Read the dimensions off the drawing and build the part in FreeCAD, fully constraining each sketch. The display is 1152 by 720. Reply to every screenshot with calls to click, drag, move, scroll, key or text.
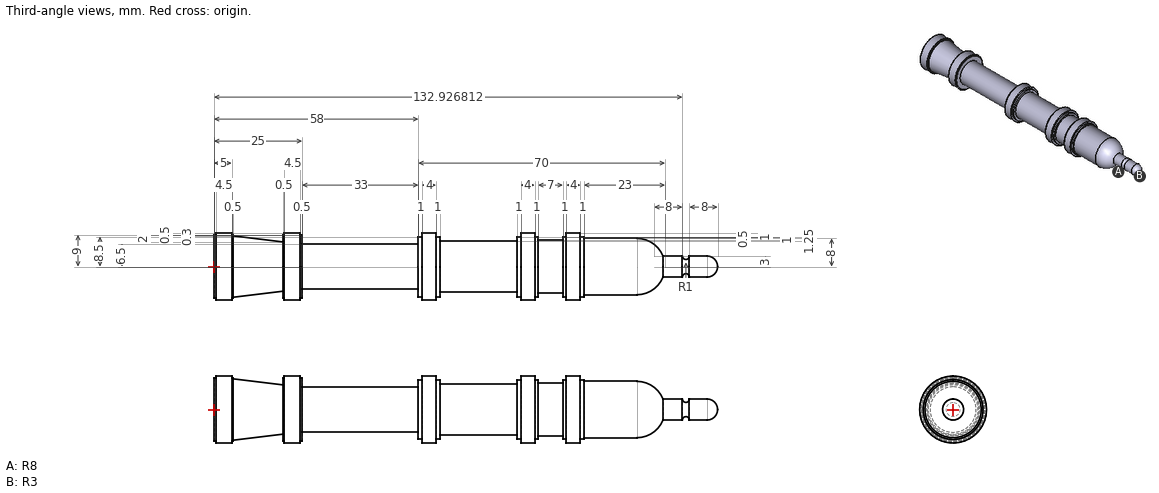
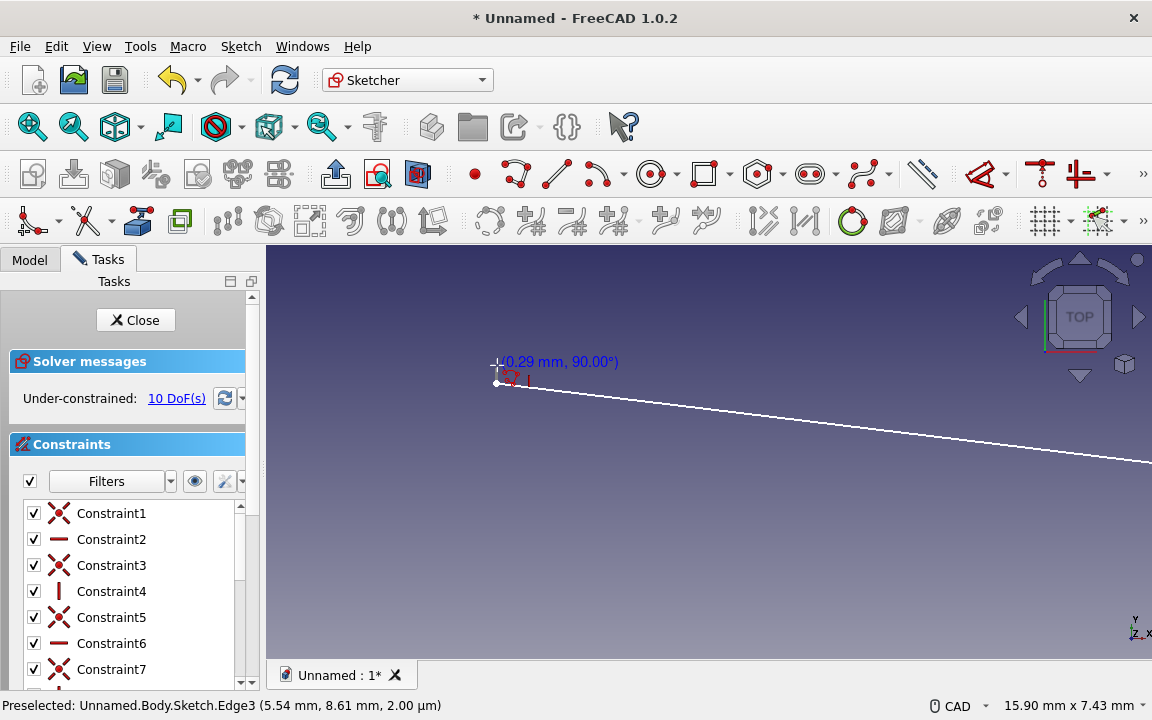
click(497, 364)
click(469, 364)
click(469, 337)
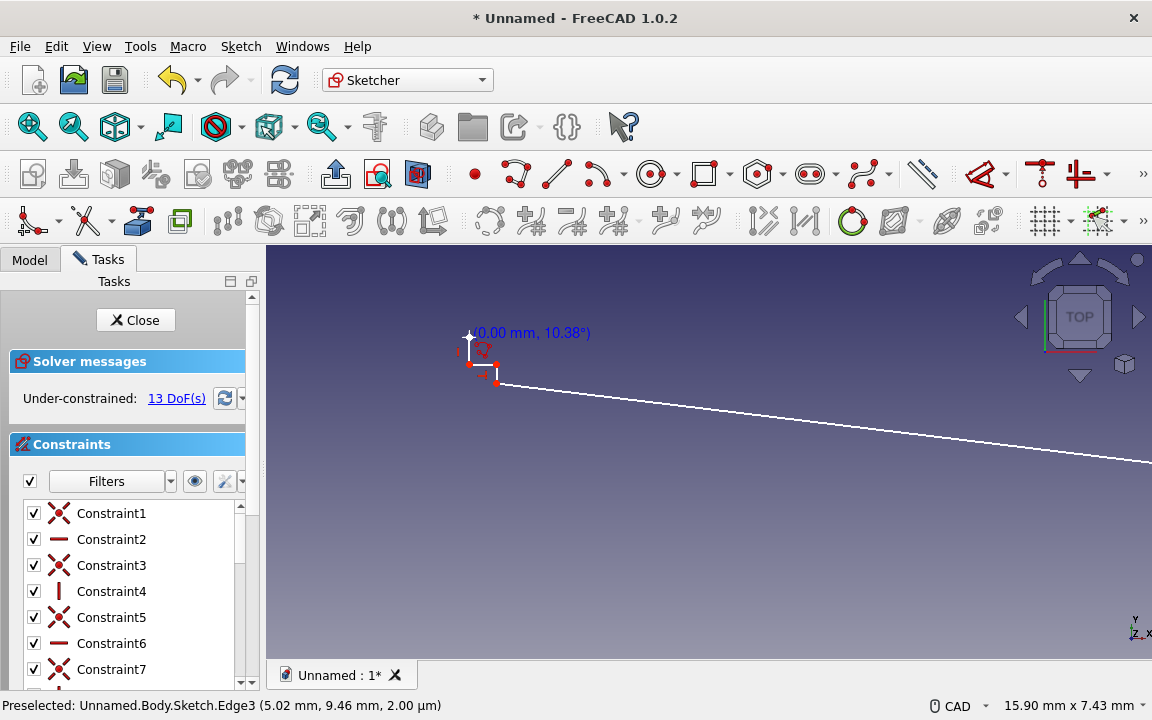
scroll(497, 365, down, 5)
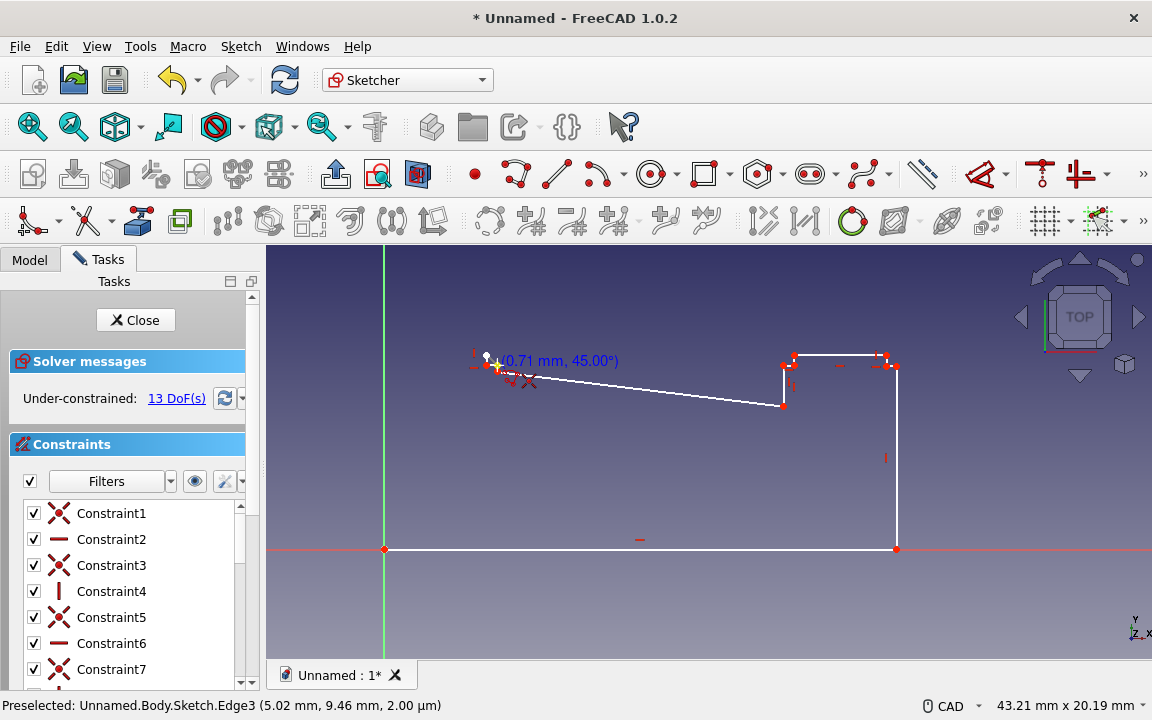
scroll(395, 355, up, 3)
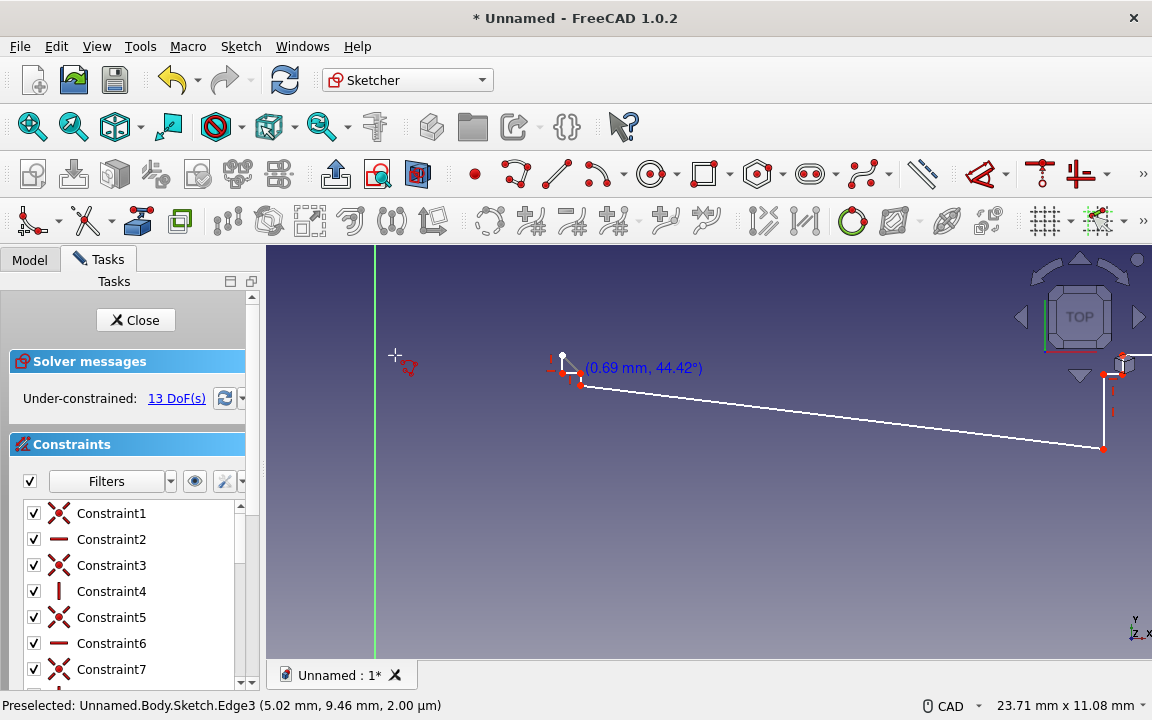
click(394, 355)
click(394, 373)
click(384, 373)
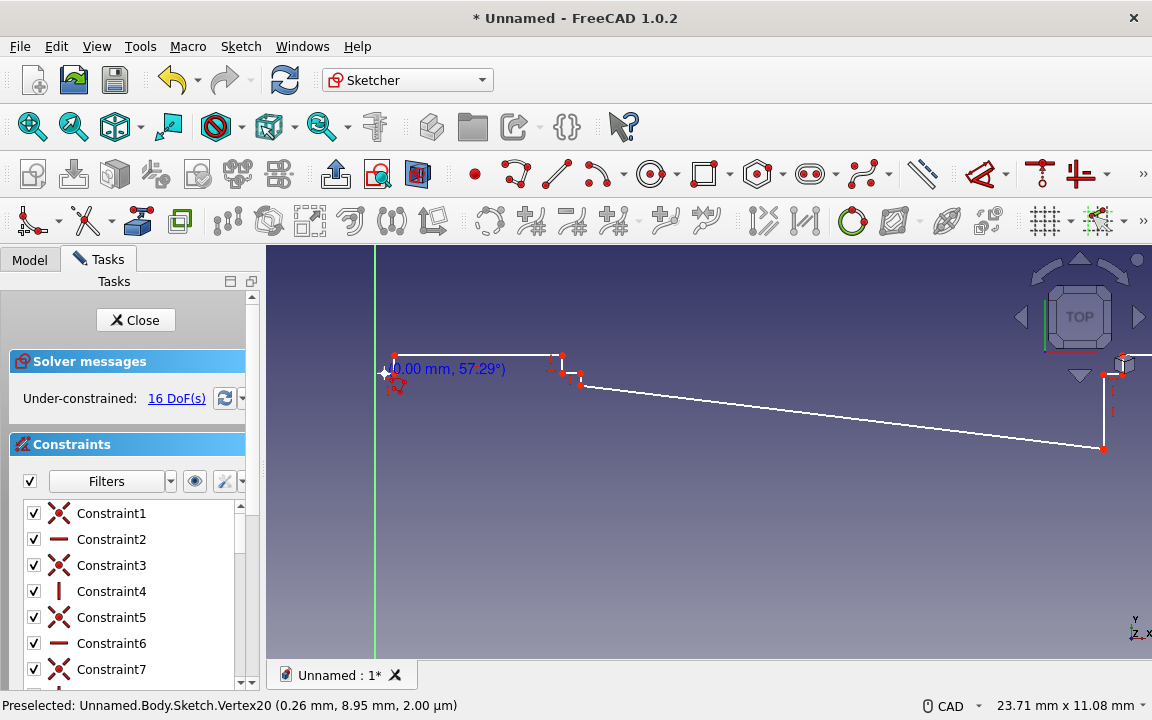
scroll(395, 355, down, 3)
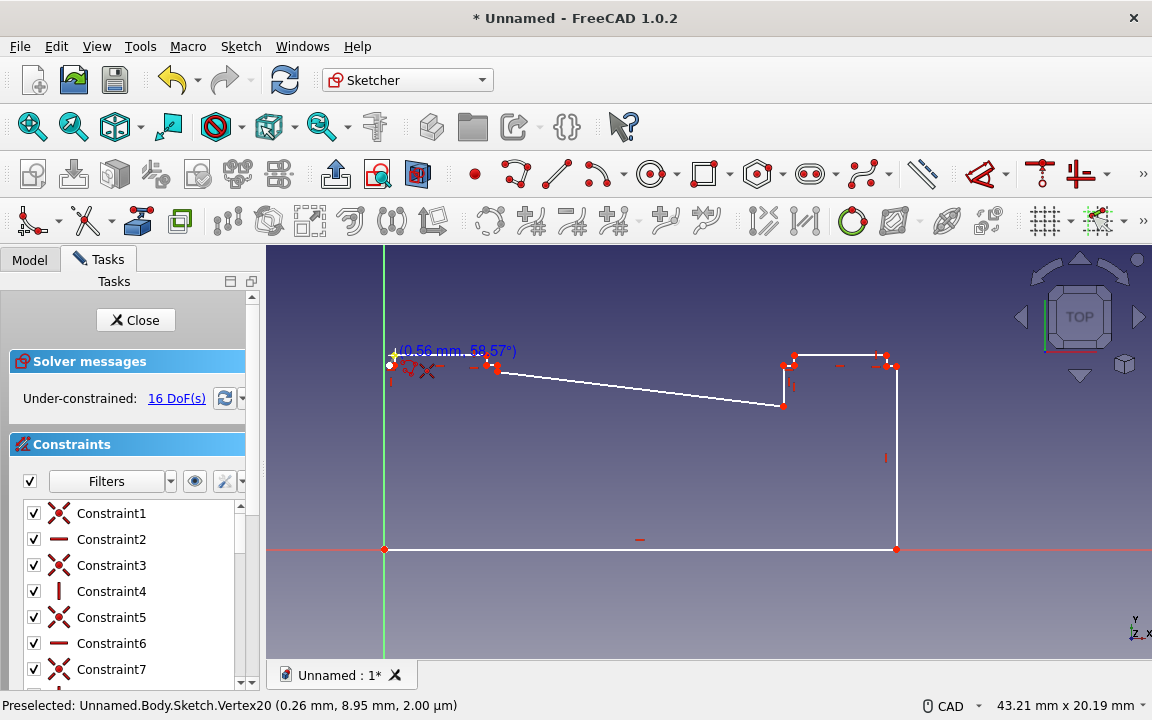
click(384, 550)
key(Escape)
key(Escape)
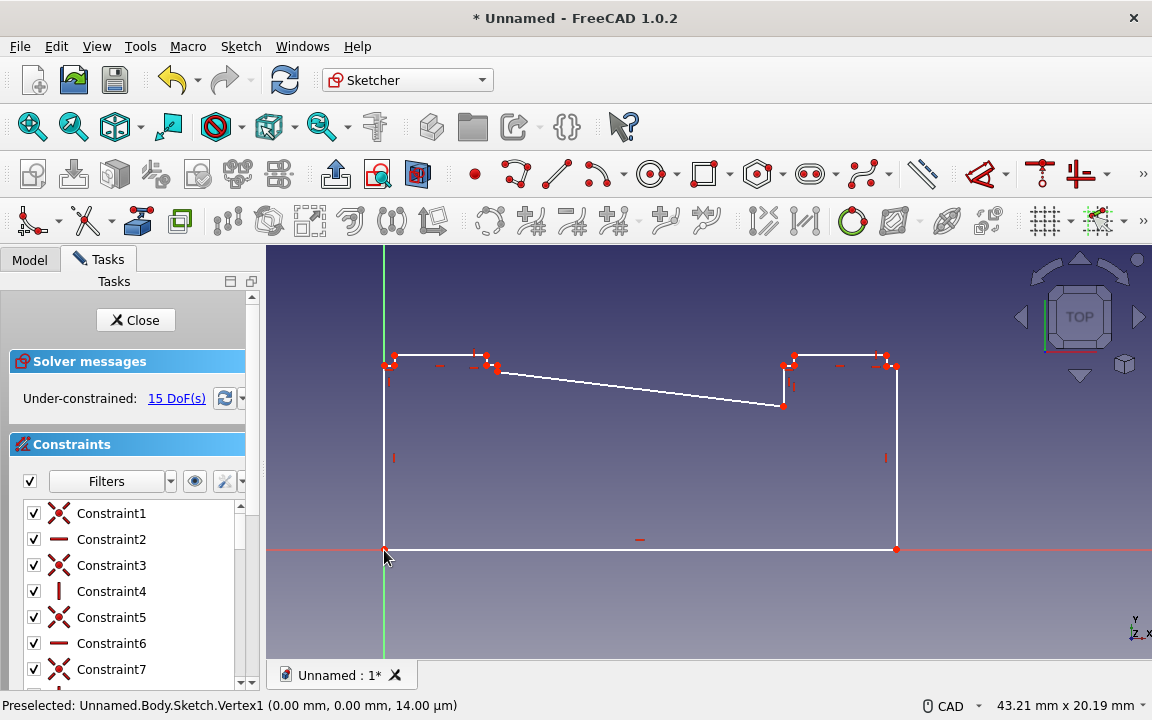
click(980, 174)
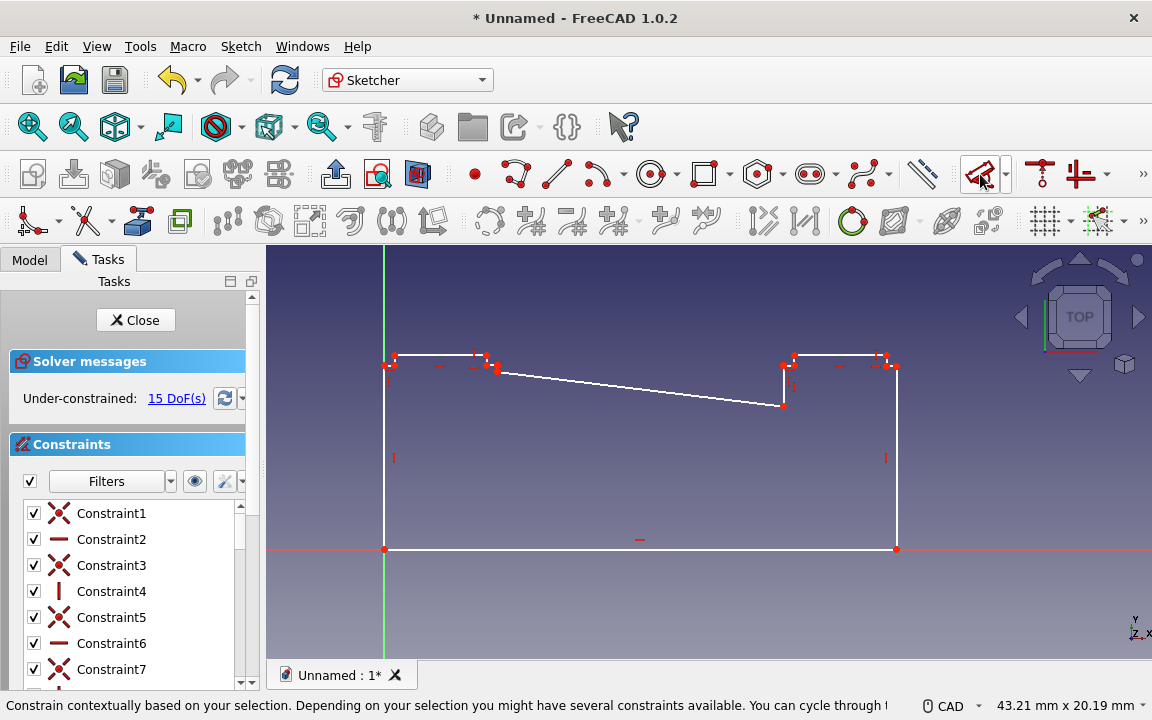
click(897, 495)
click(931, 458)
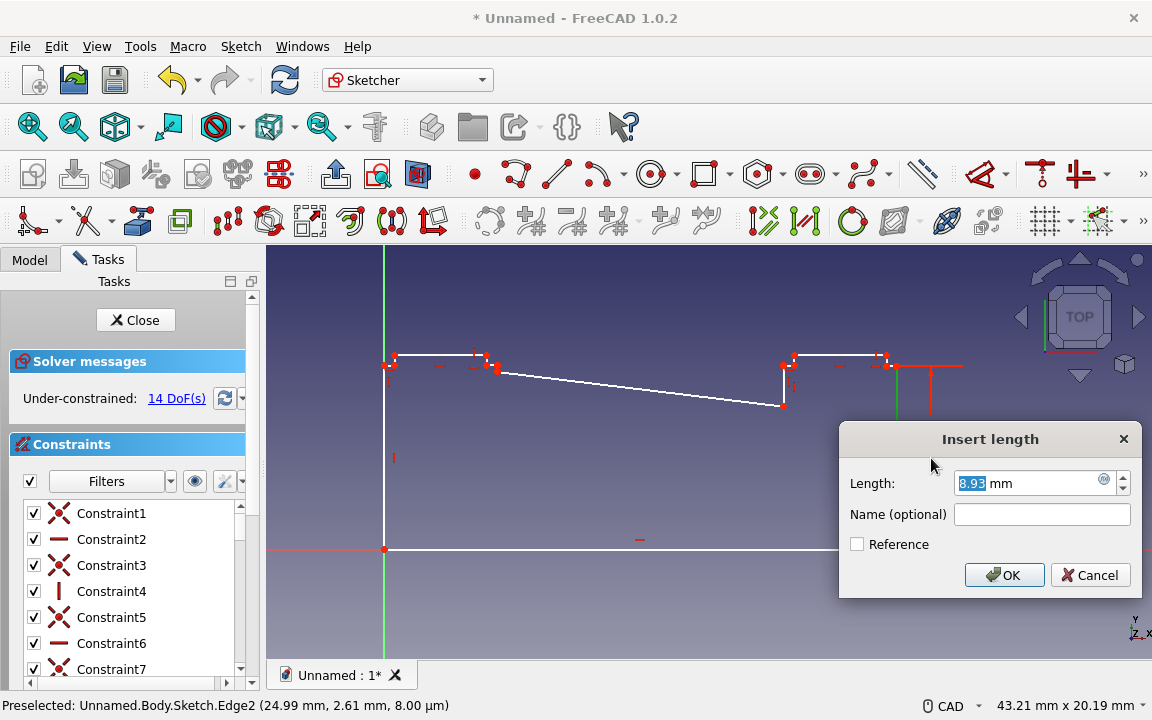
text(9)
key(Return)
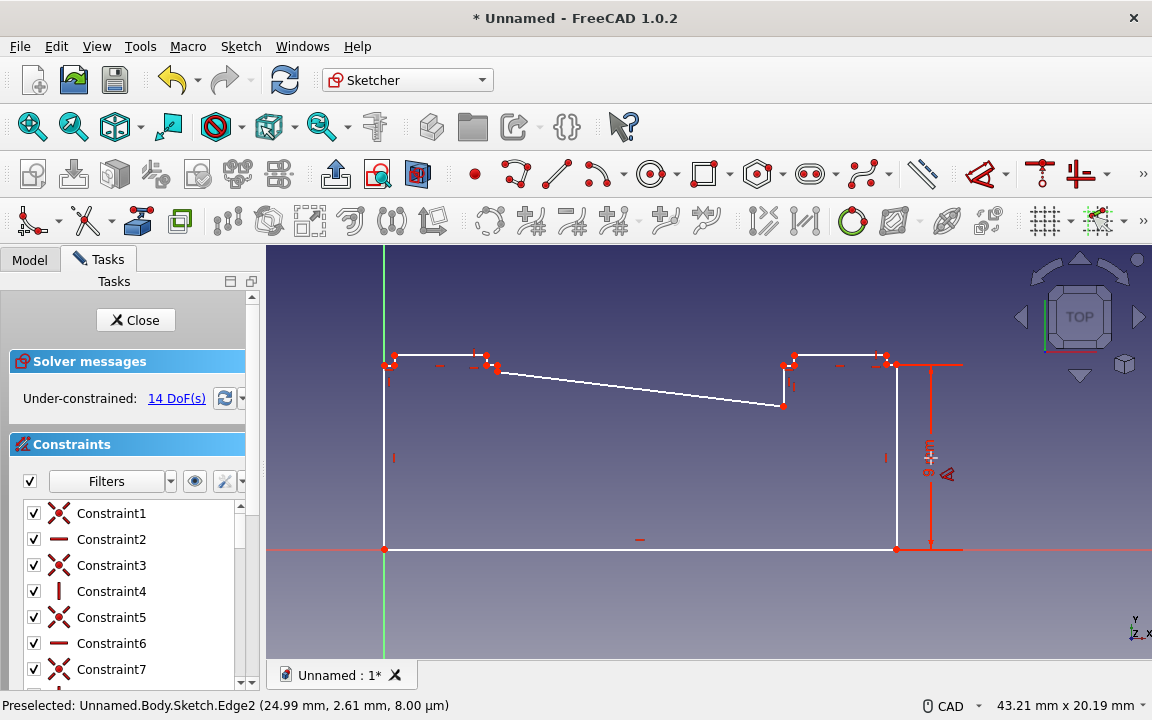
click(784, 378)
click(818, 386)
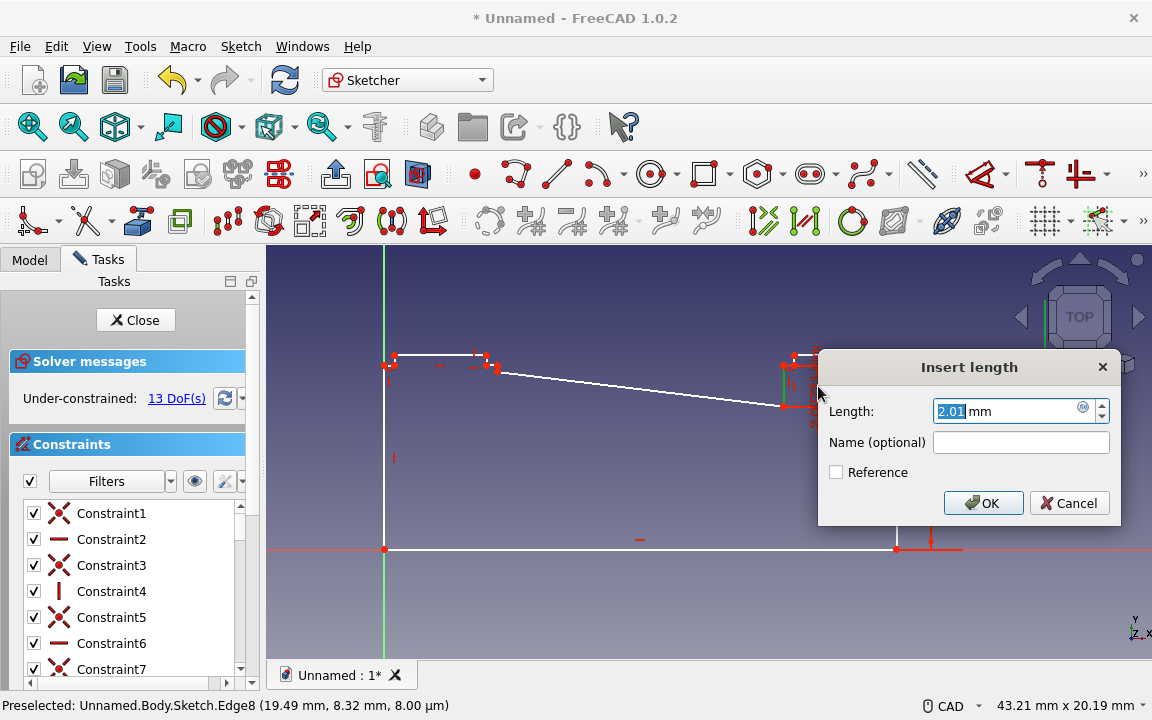
text(2)
key(Return)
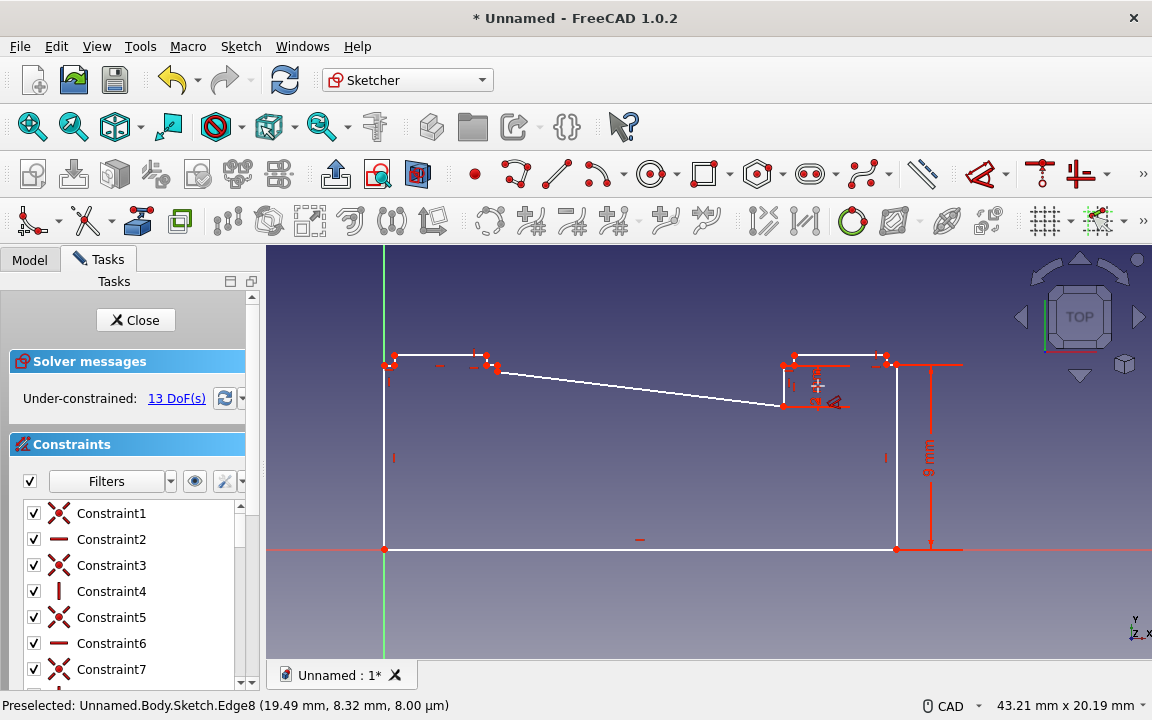
click(384, 421)
click(350, 458)